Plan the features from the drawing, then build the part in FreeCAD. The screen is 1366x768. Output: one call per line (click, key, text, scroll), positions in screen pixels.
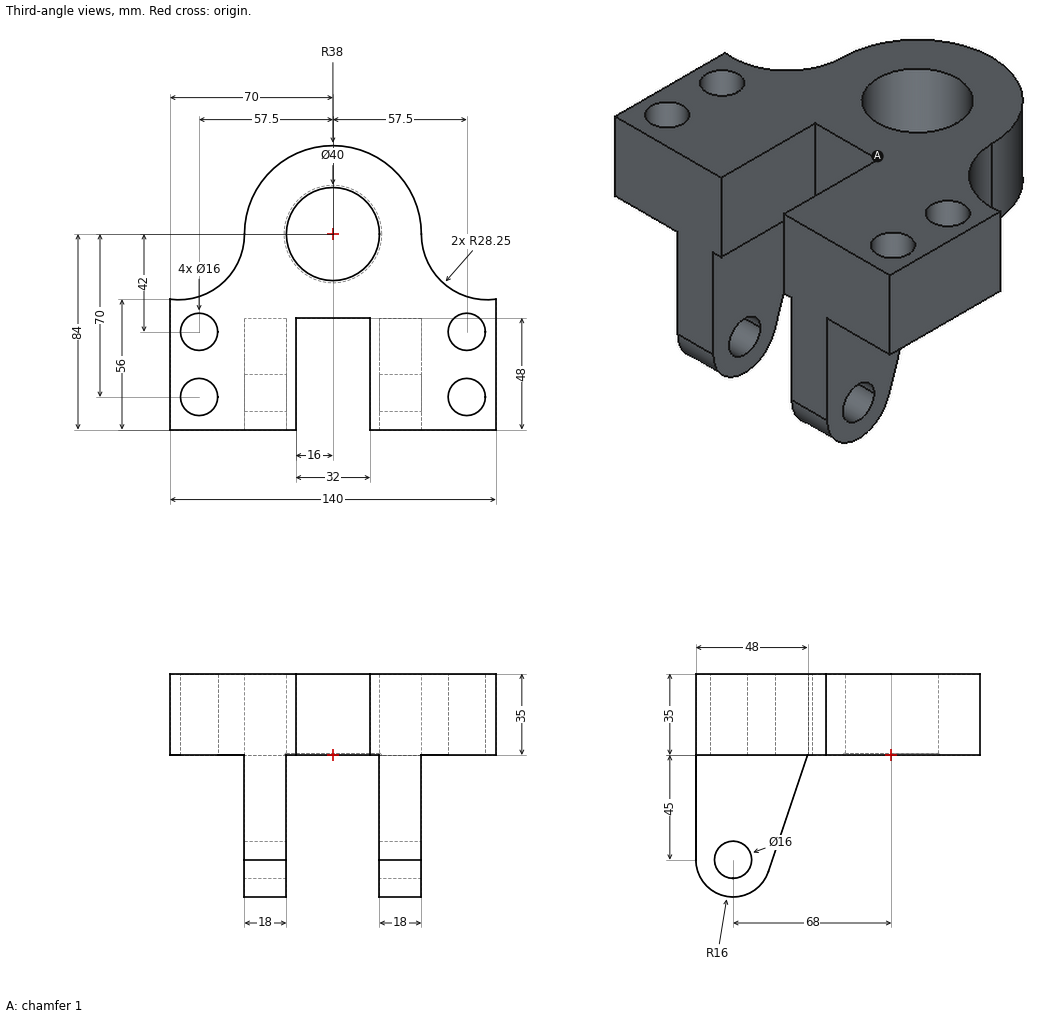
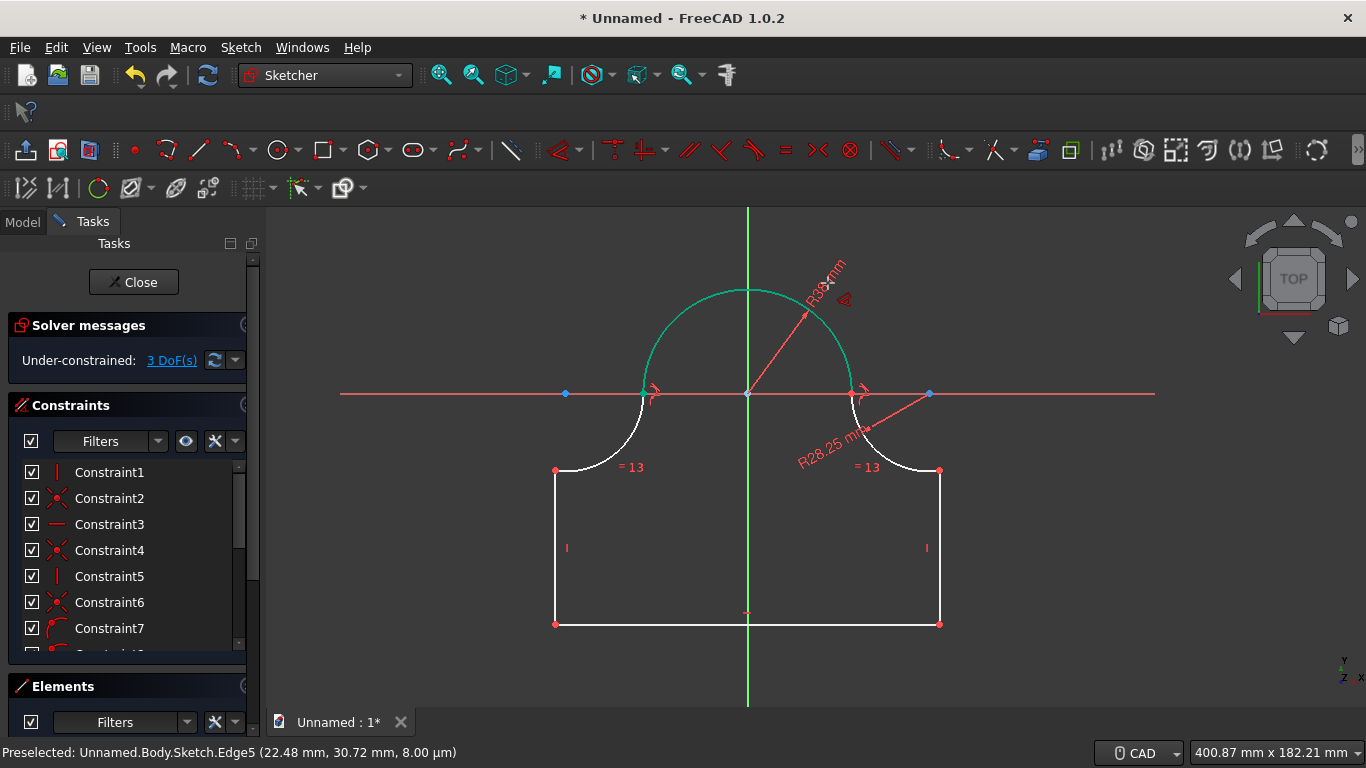
click(555, 517)
click(521, 548)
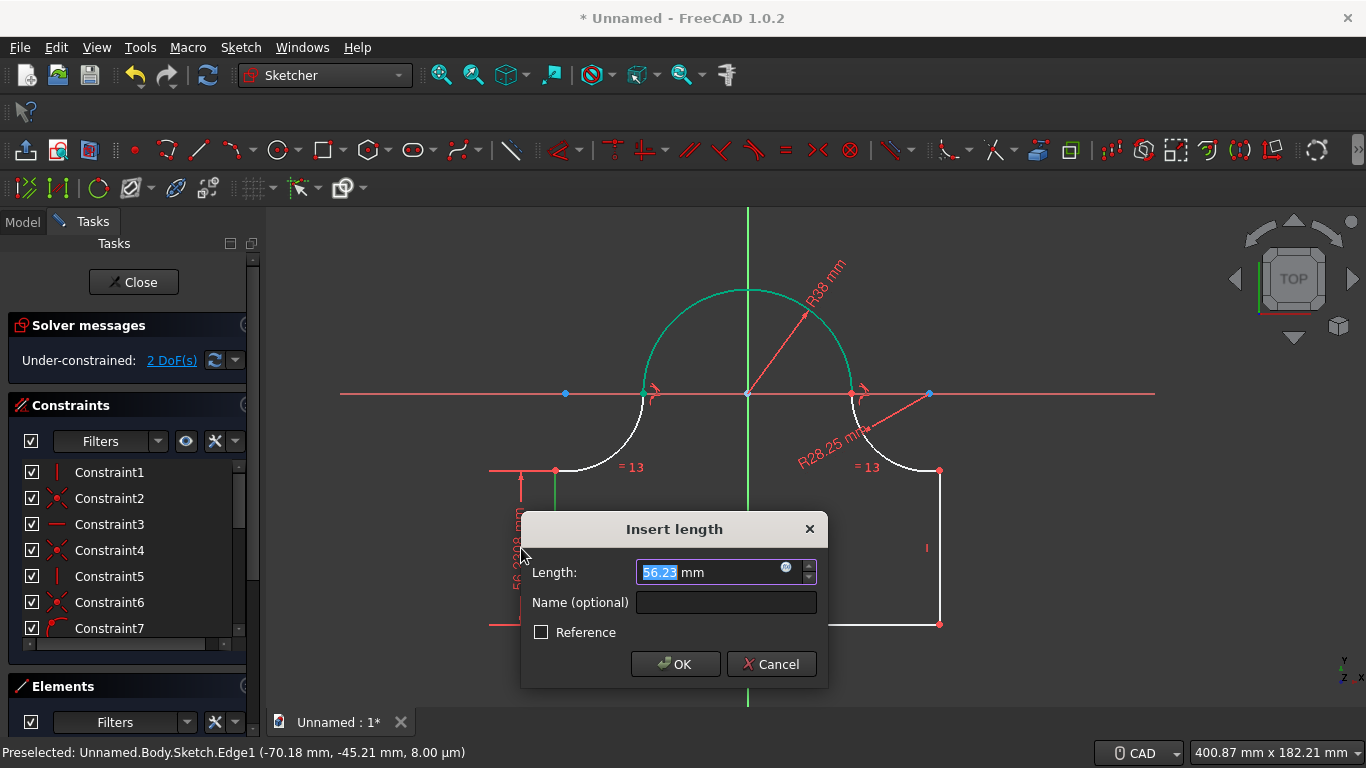
text(56)
key(Return)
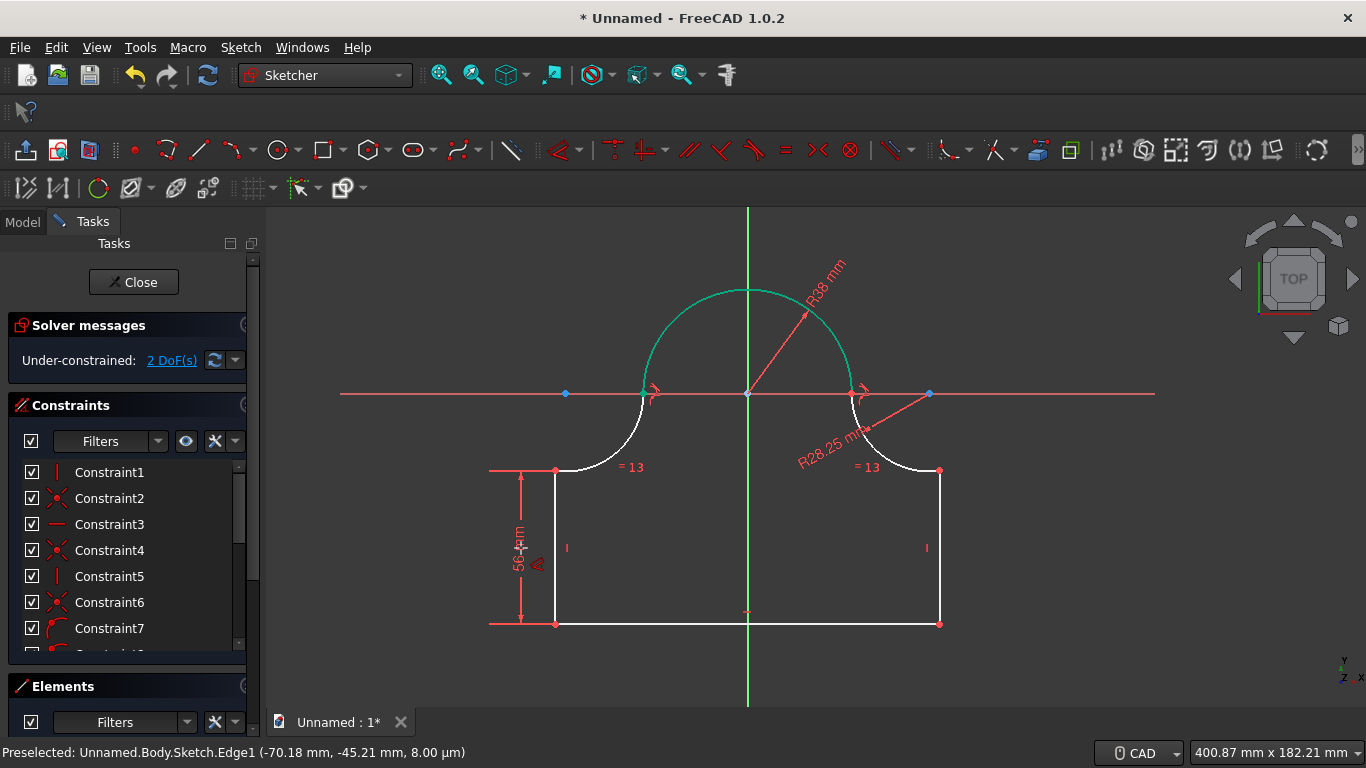
click(671, 624)
click(659, 658)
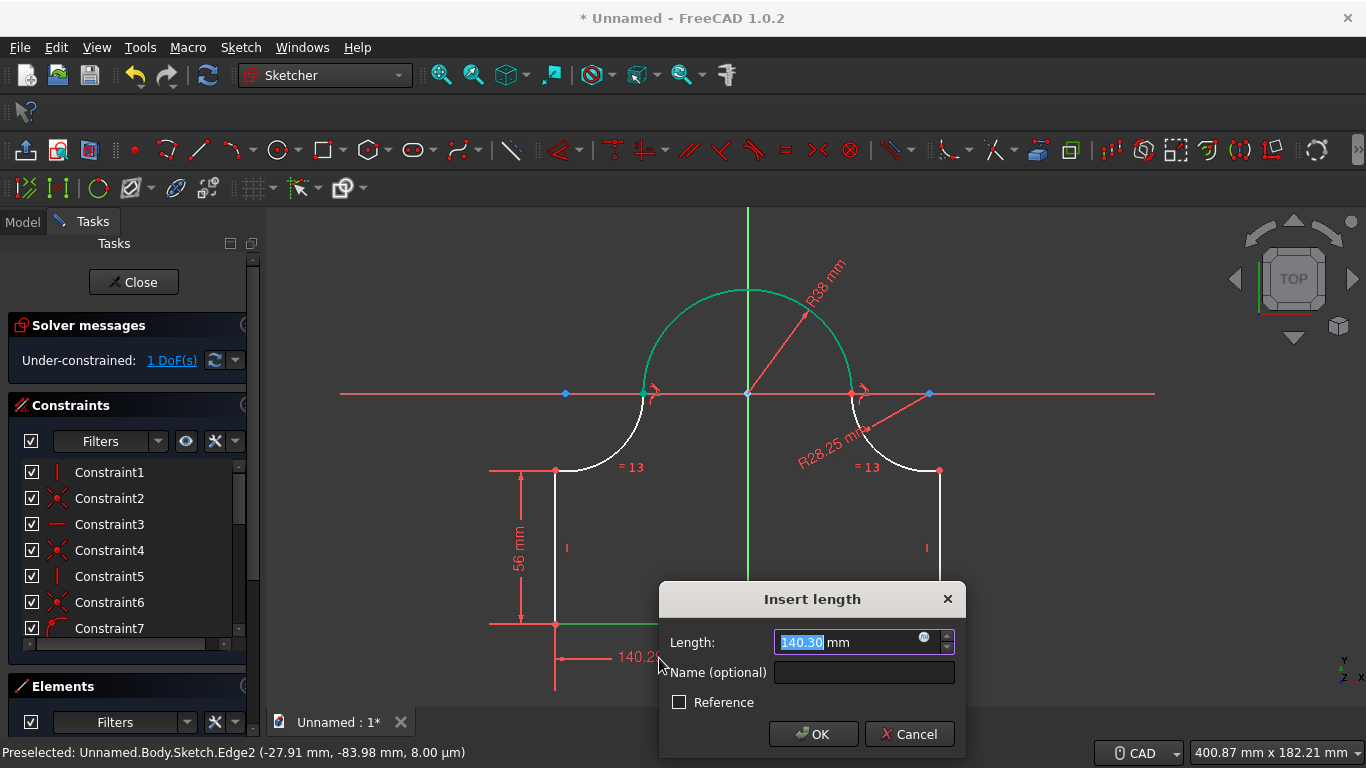
text(140)
key(Return)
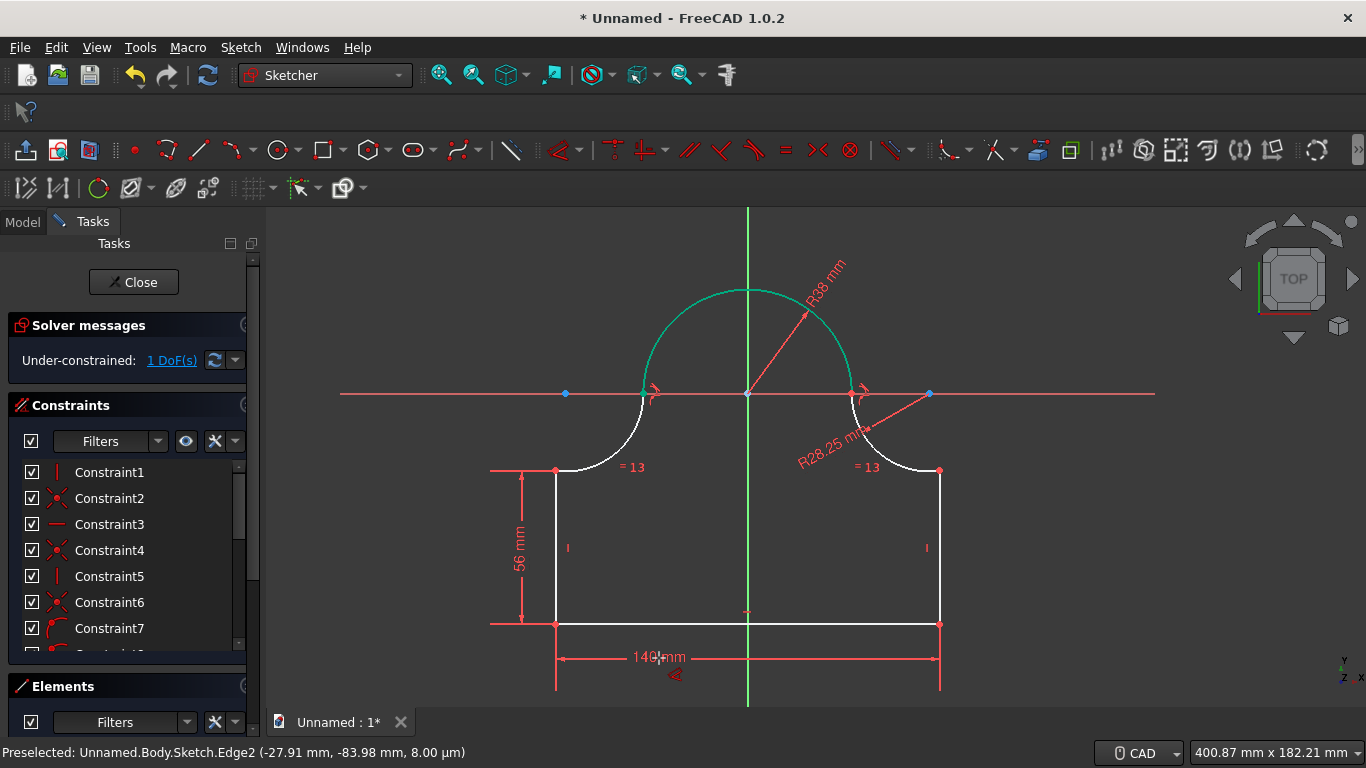
click(556, 471)
click(607, 360)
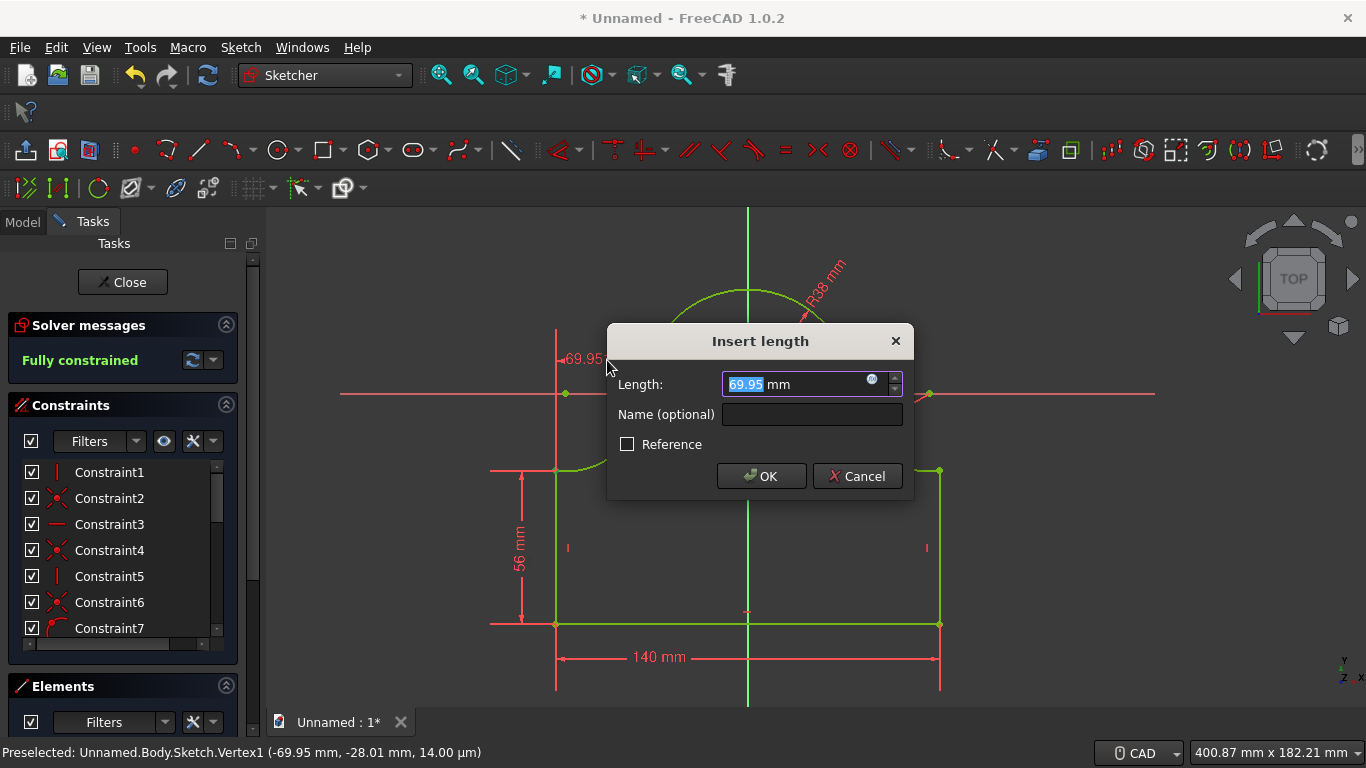
text(70)
key(Return)
key(Escape)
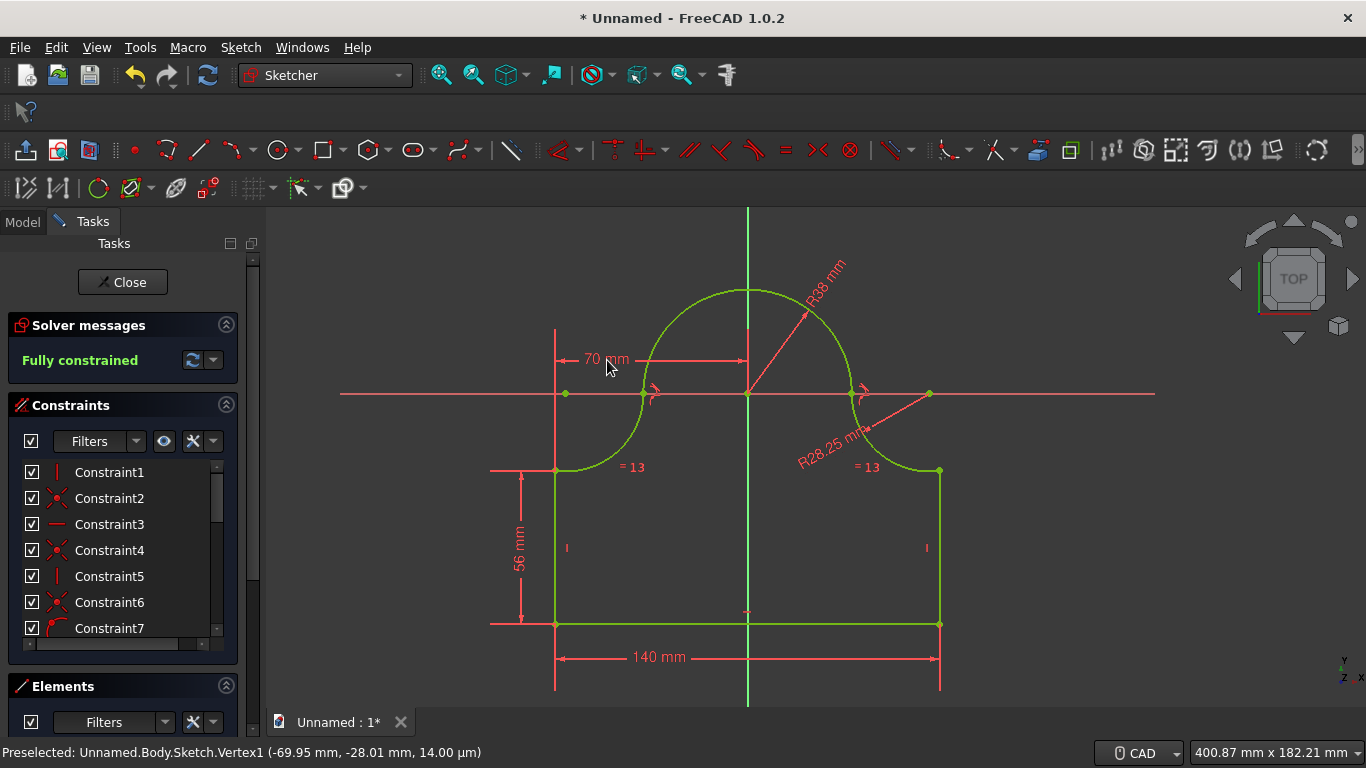
click(123, 282)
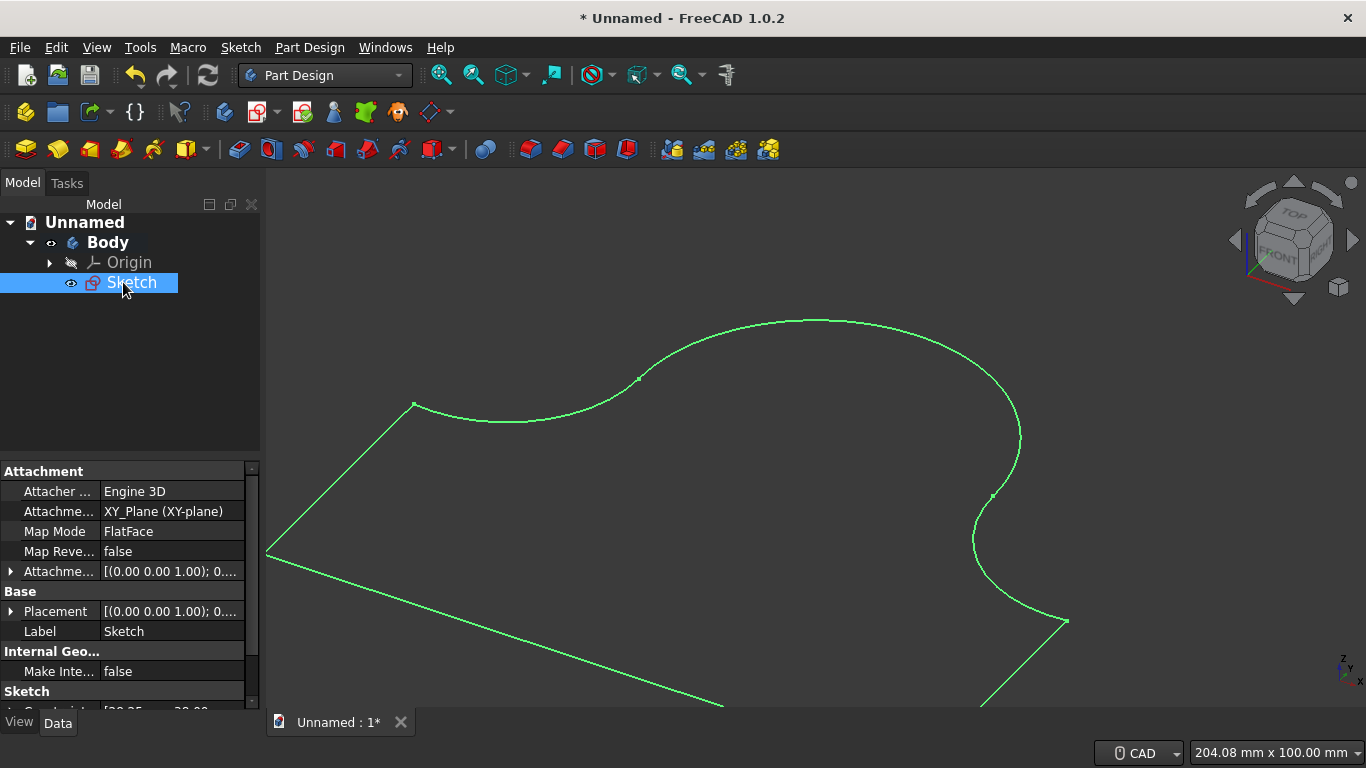
click(26, 150)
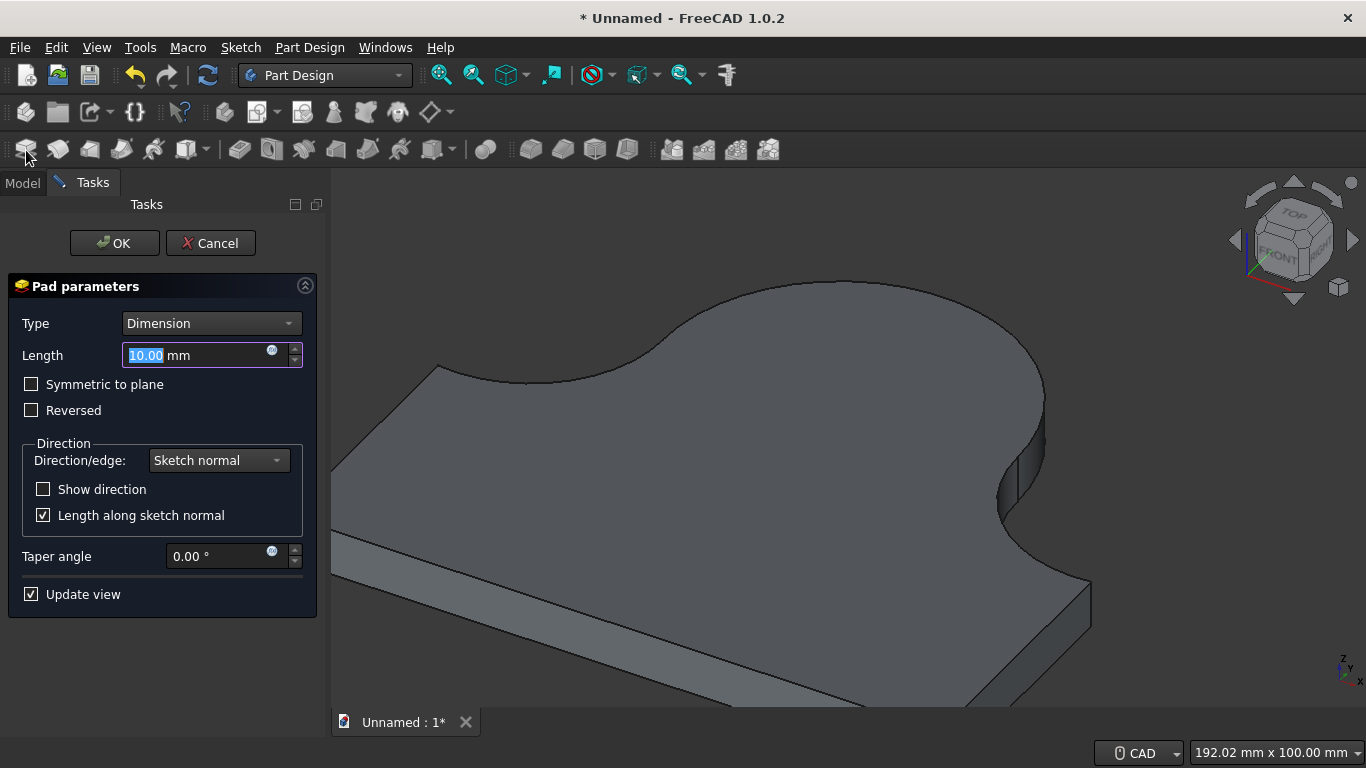
text(35)
key(Tab)